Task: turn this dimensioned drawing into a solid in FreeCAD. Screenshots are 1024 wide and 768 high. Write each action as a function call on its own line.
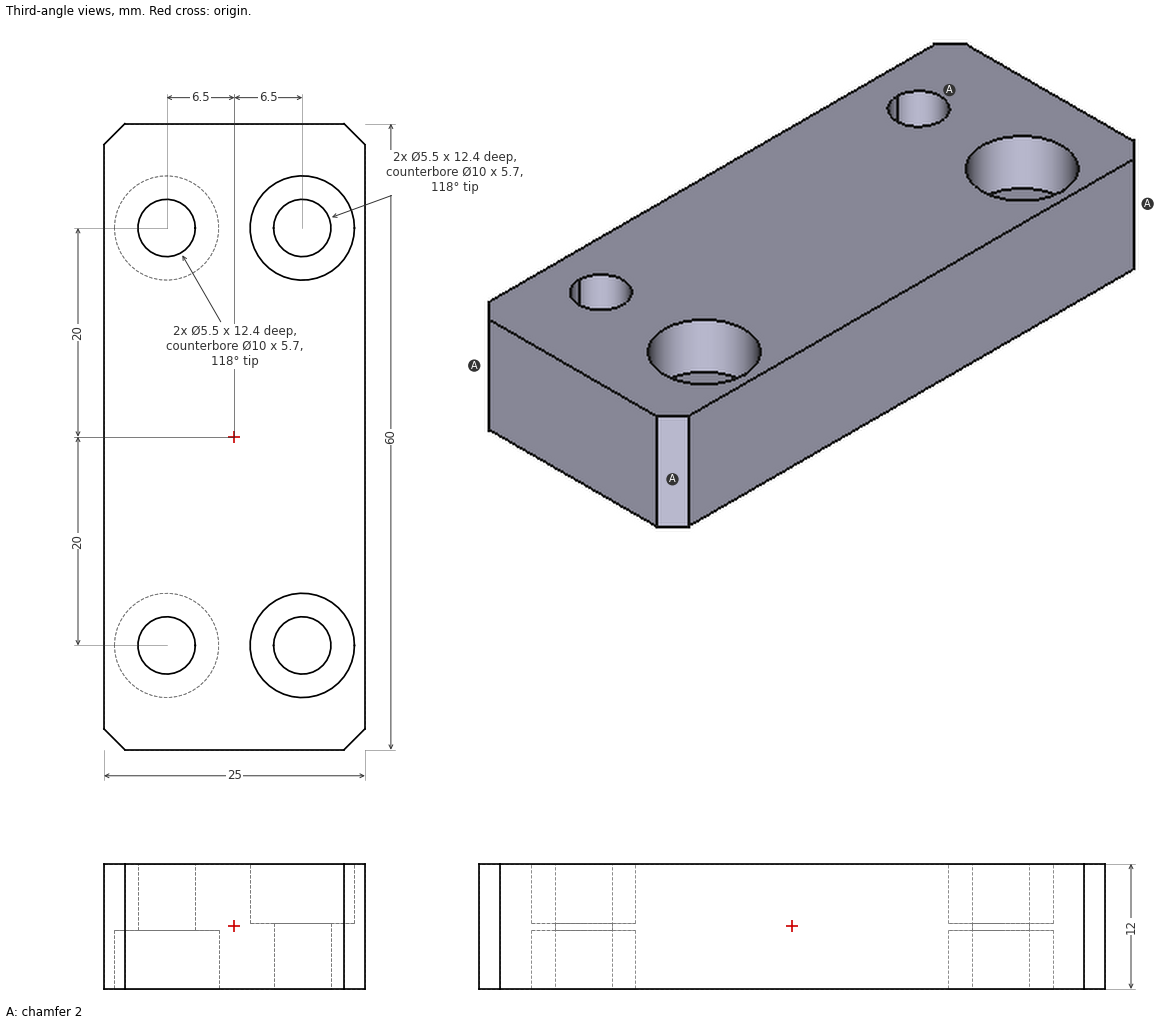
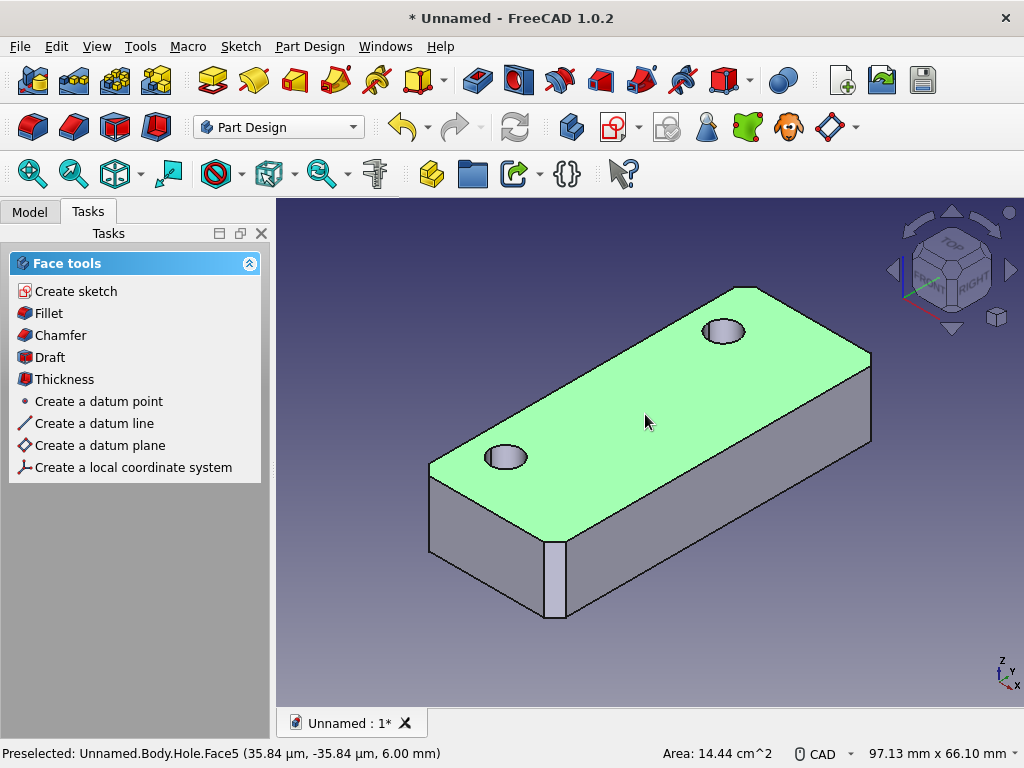
click(612, 128)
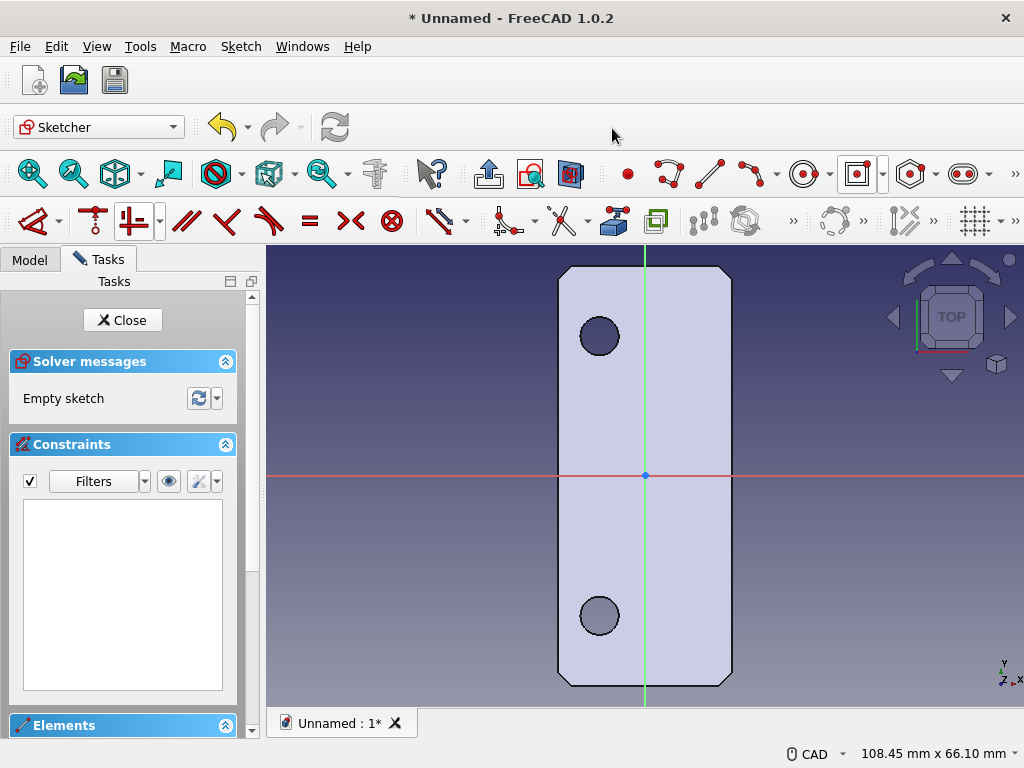
click(804, 174)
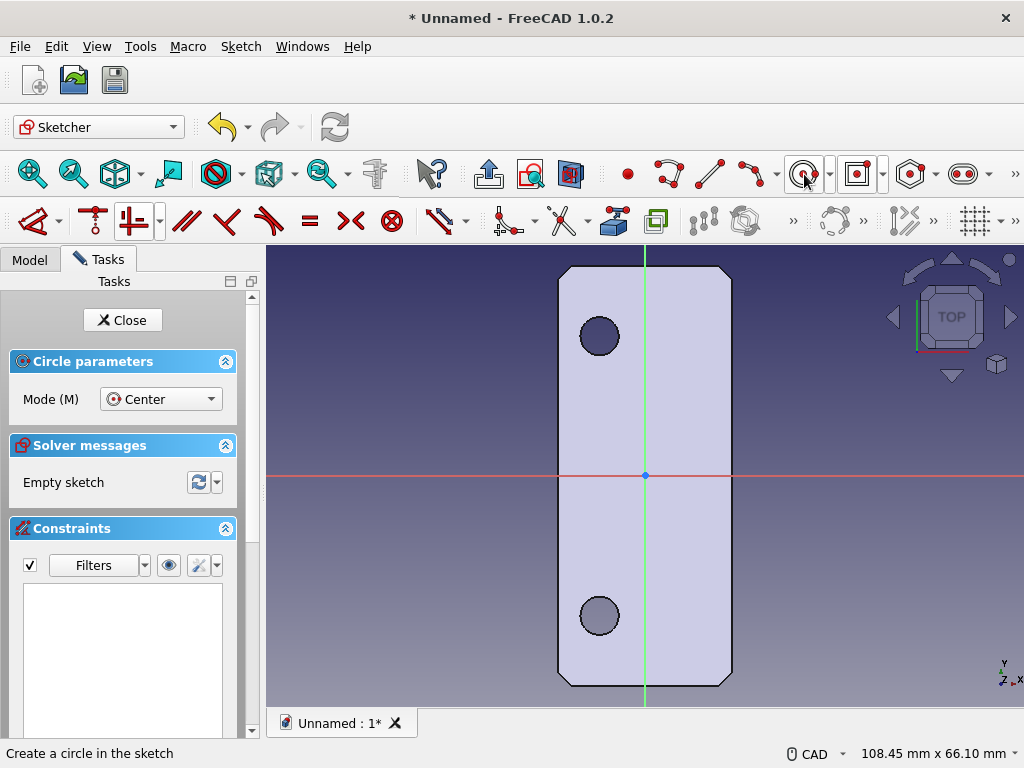
click(690, 336)
click(704, 323)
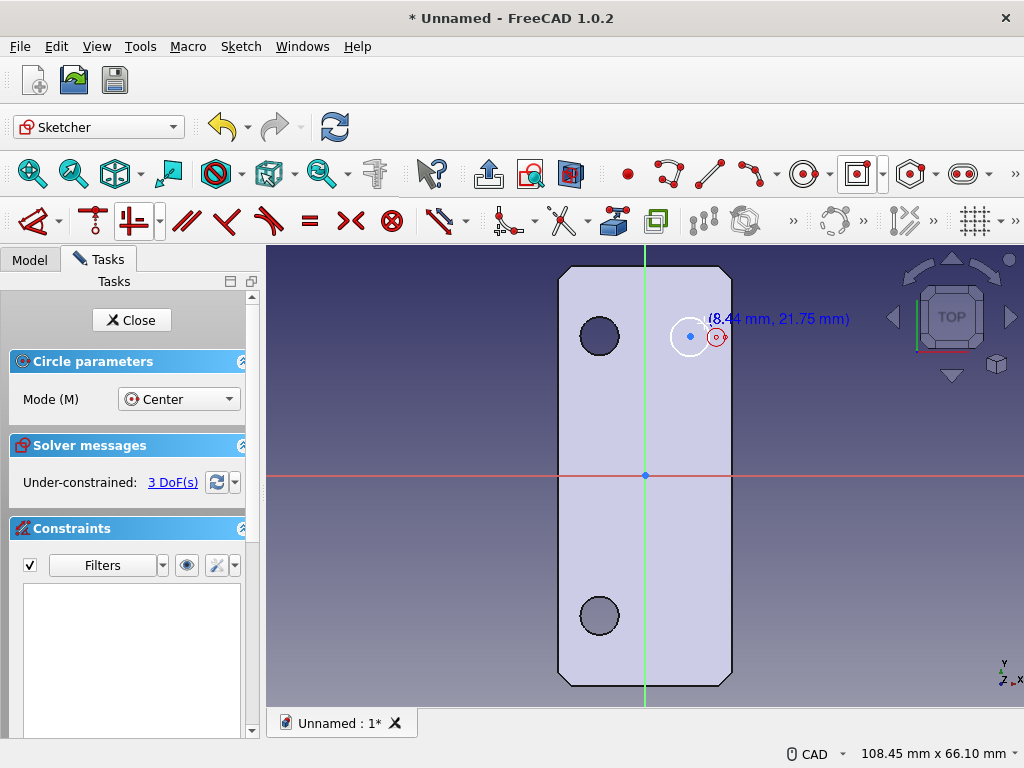
click(690, 616)
click(704, 602)
key(Escape)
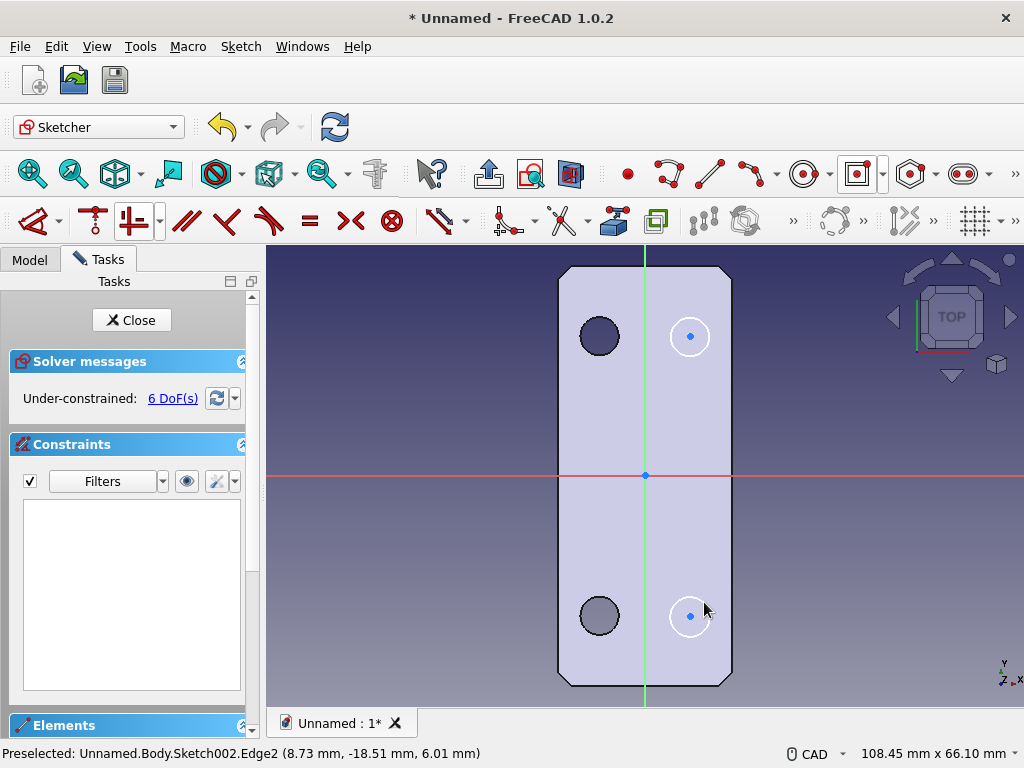
click(703, 323)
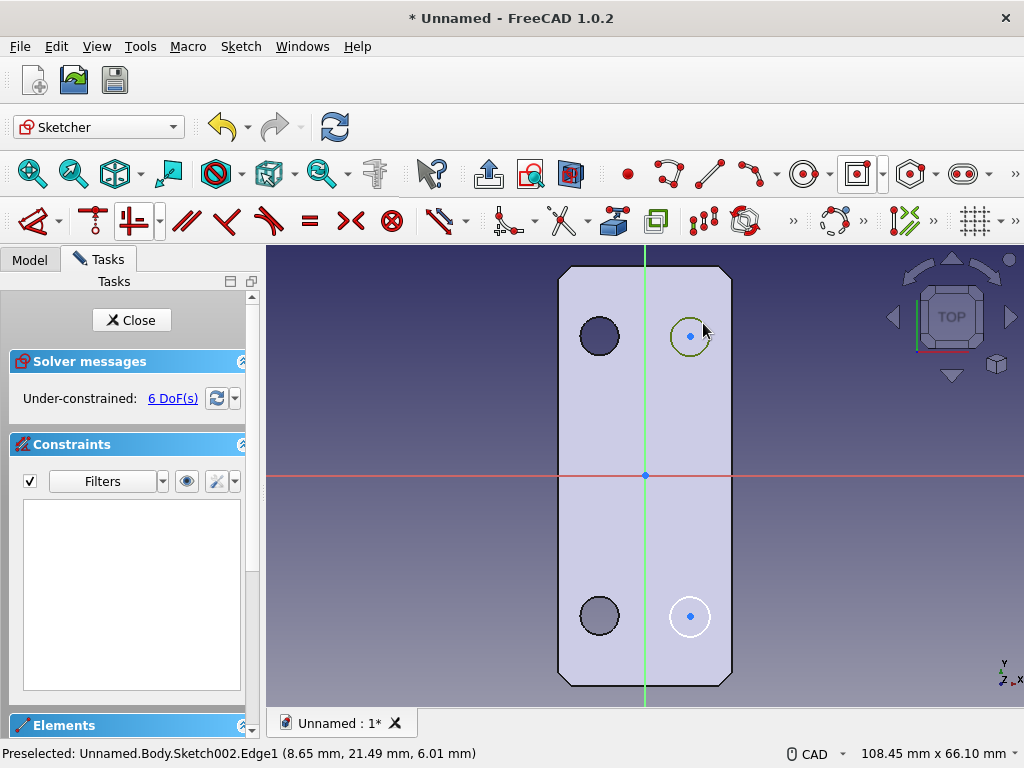
click(704, 603)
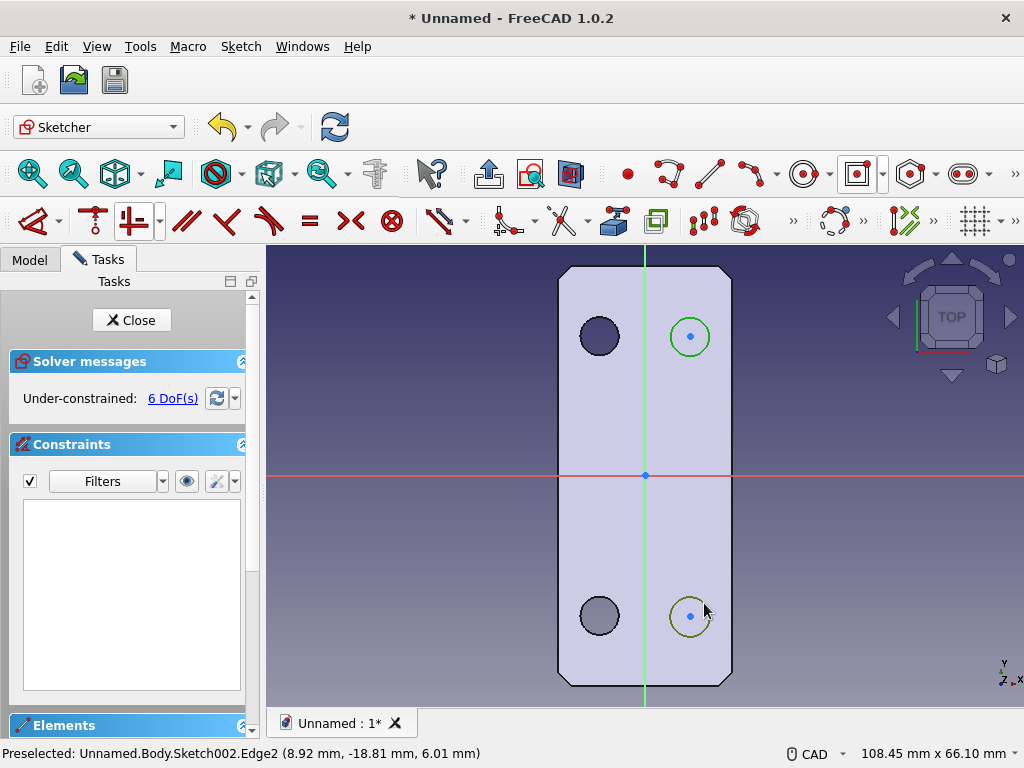
click(310, 222)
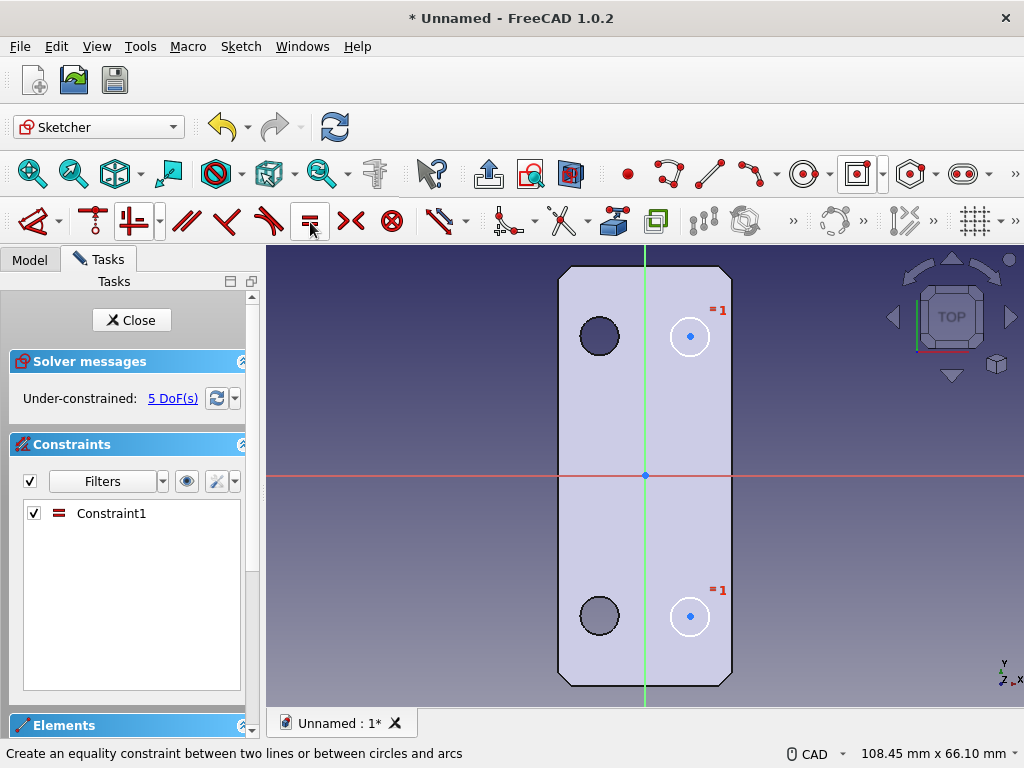
click(690, 337)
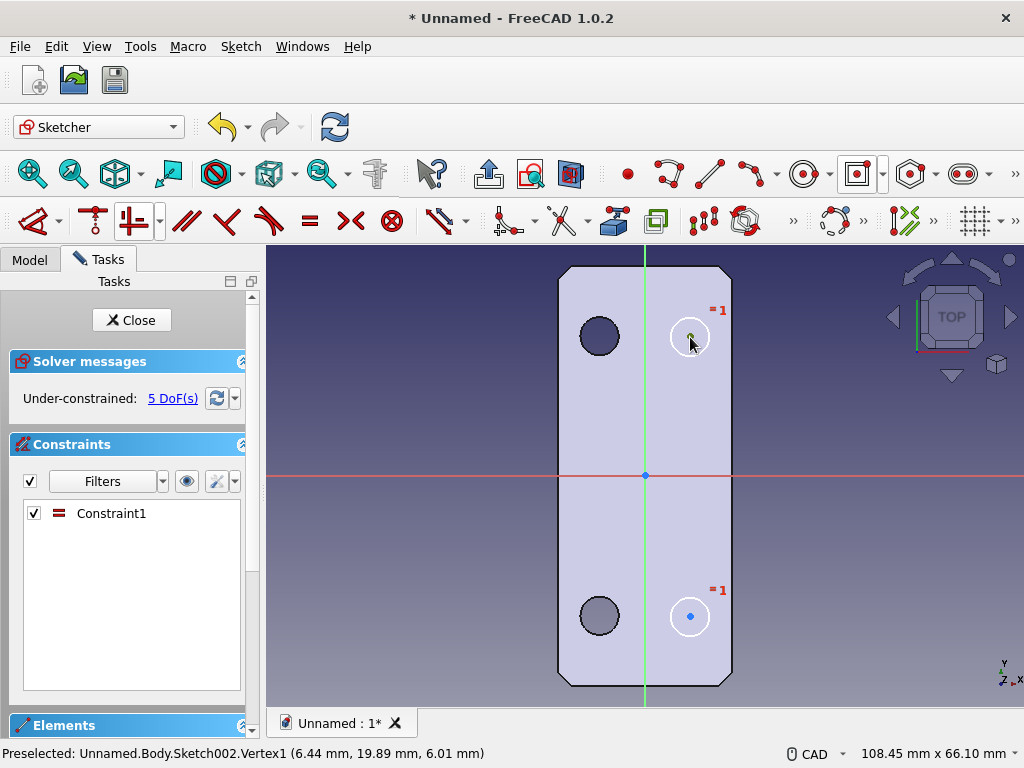
click(690, 617)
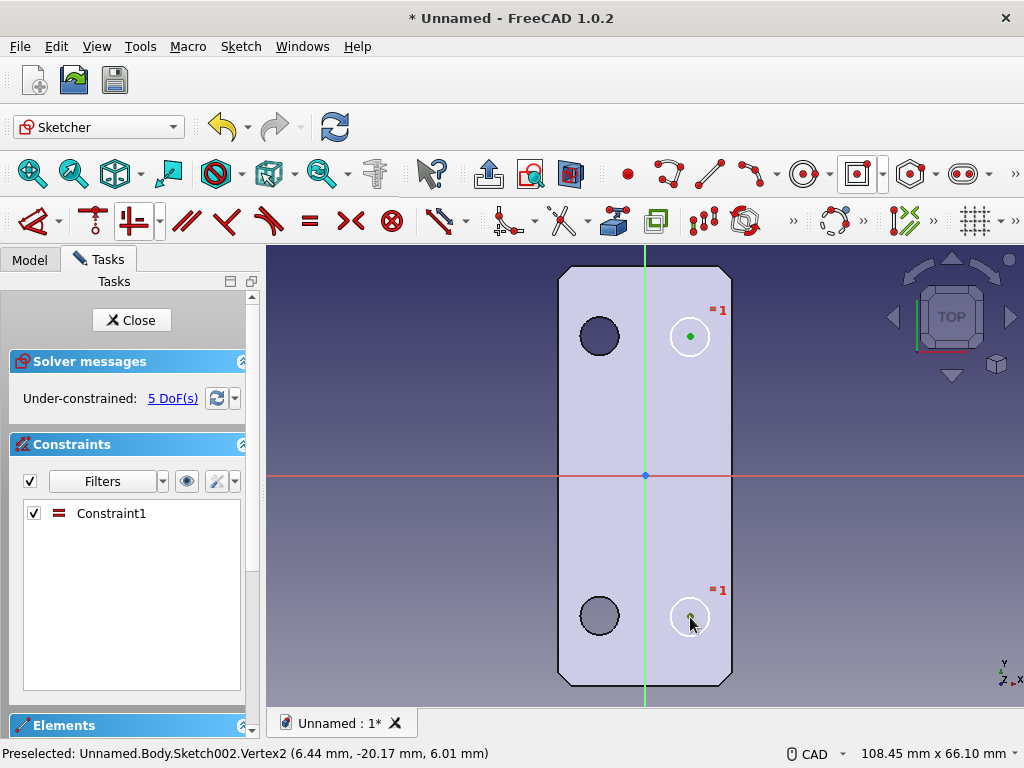
click(160, 222)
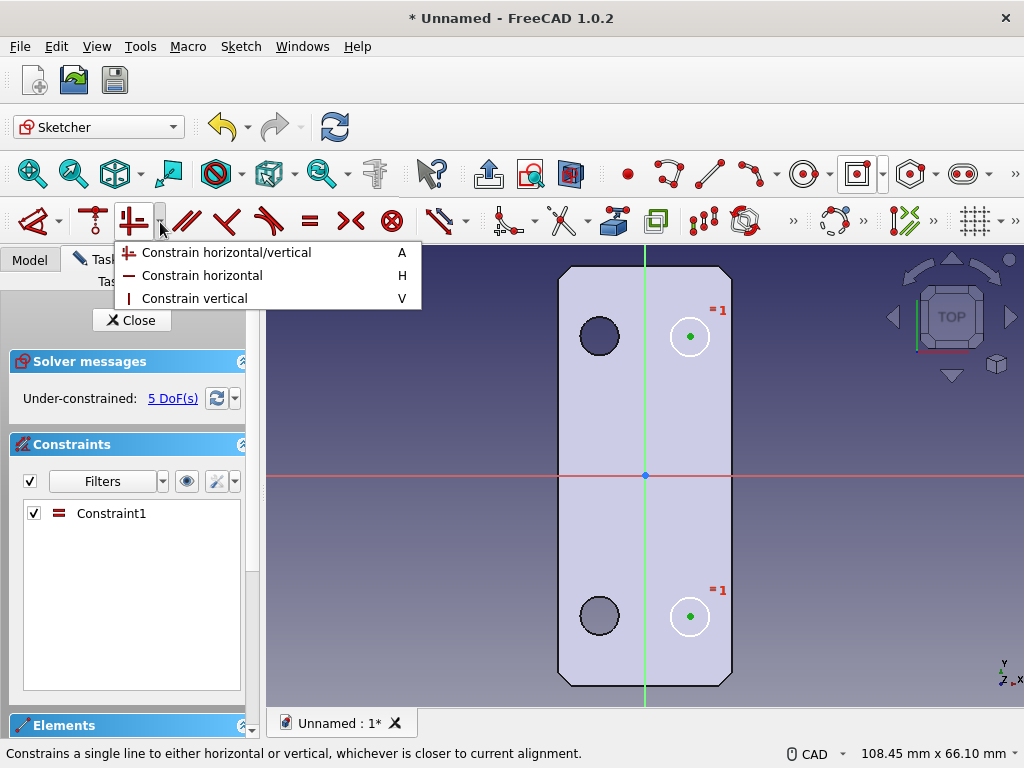
click(268, 298)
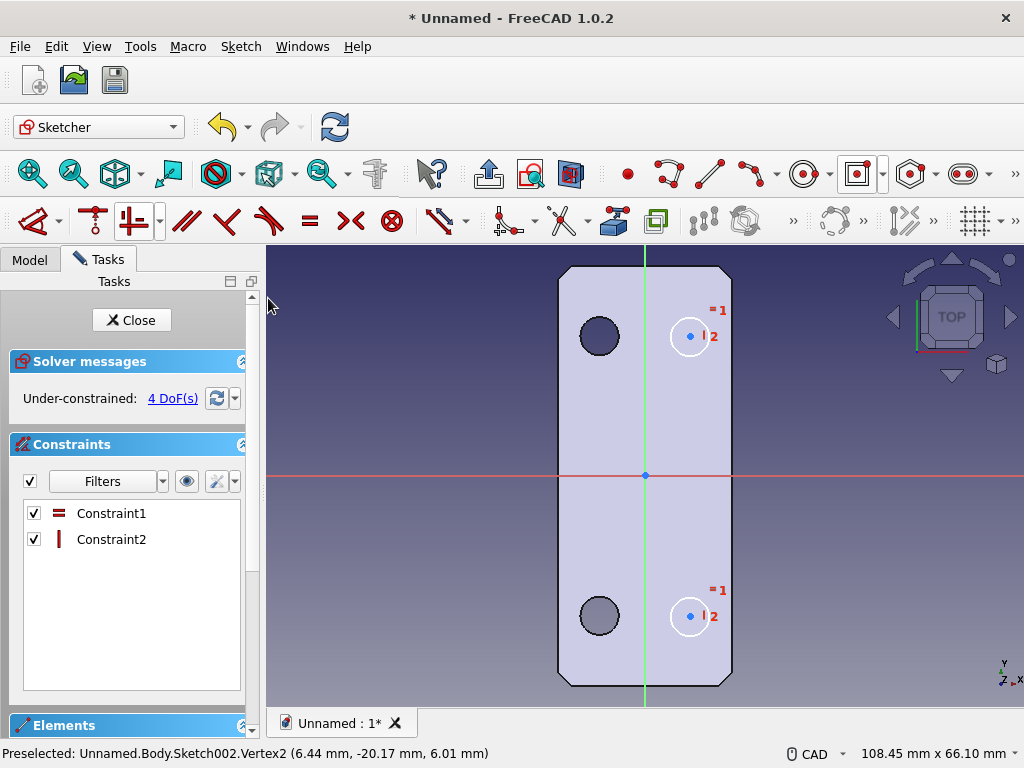
click(32, 222)